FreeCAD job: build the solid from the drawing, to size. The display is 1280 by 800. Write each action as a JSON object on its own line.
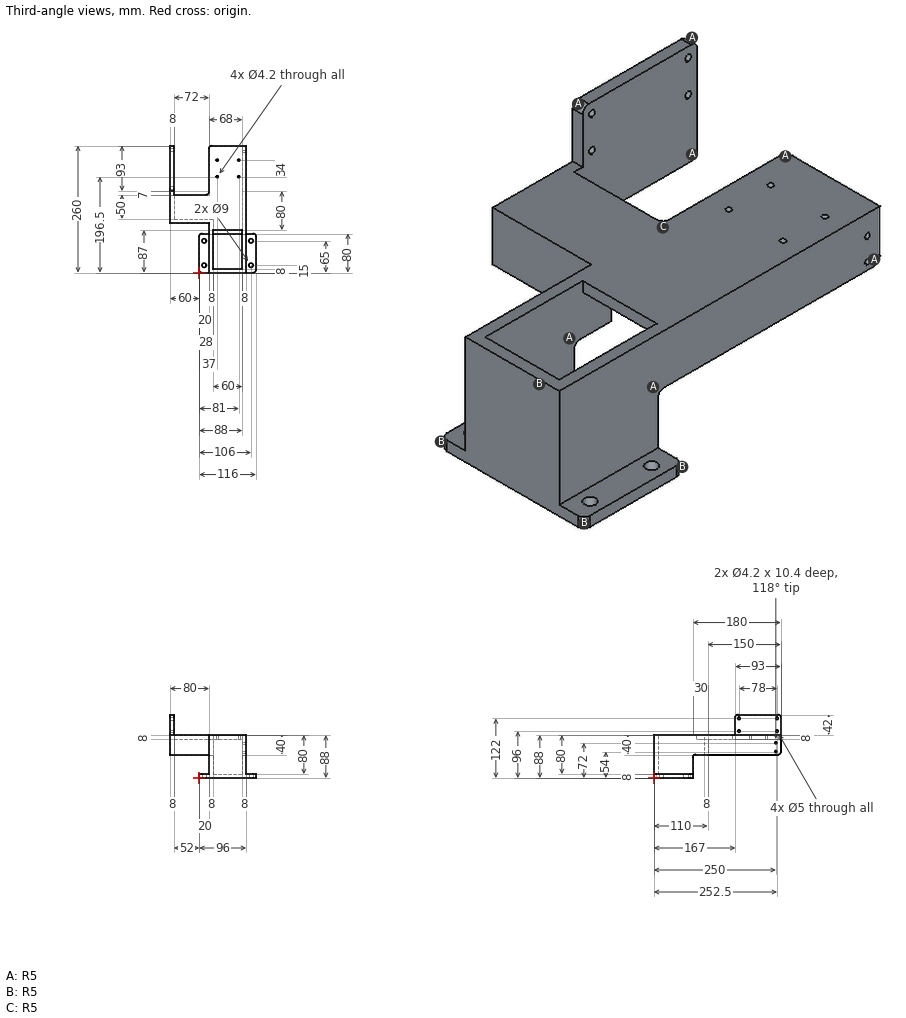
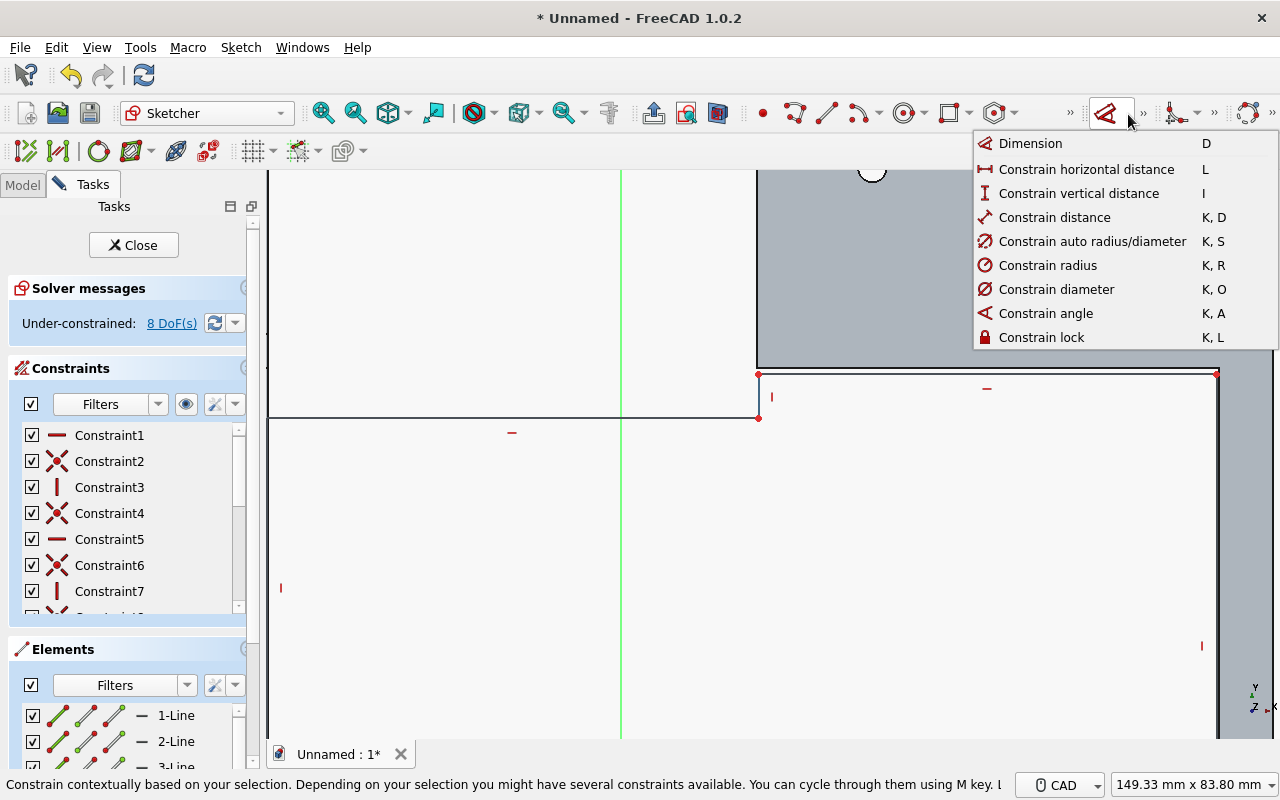
{"action": "left_click", "coordinate": [1126, 193]}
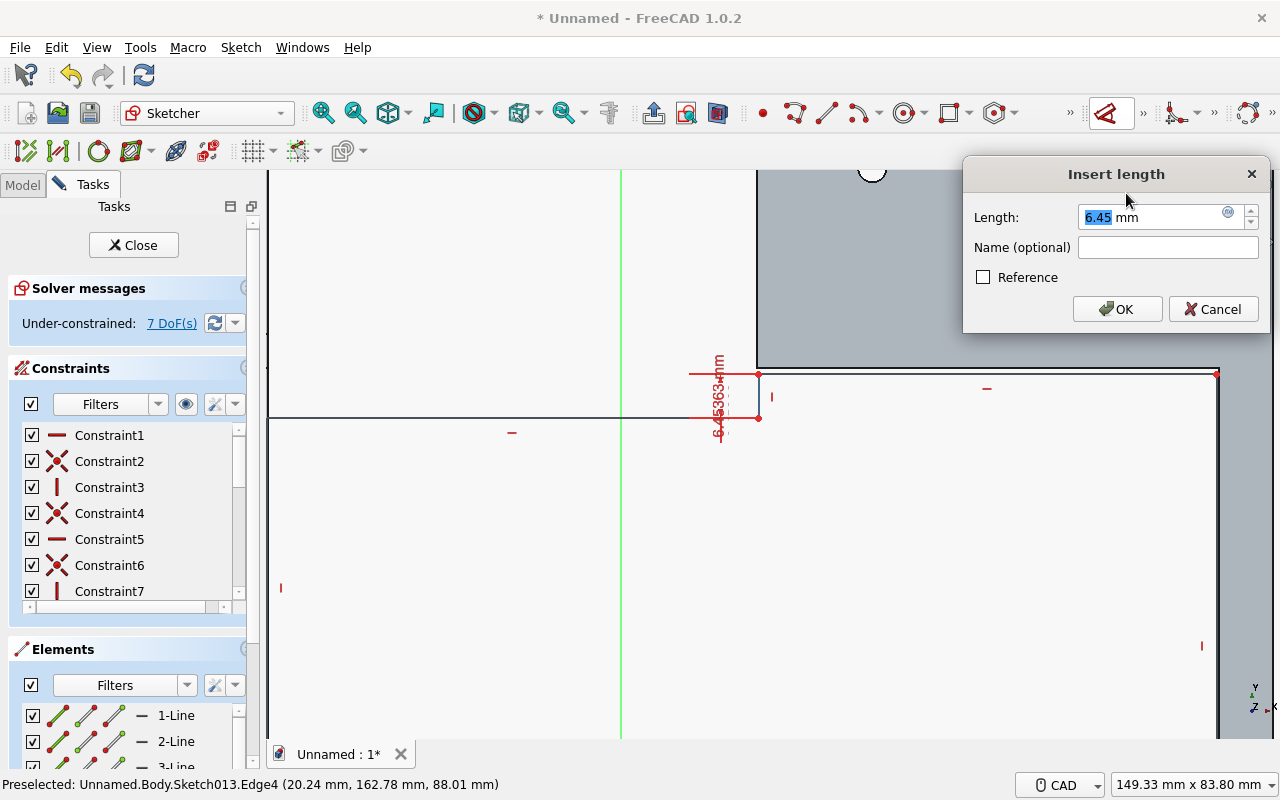
{"action": "type", "text": "7"}
{"action": "key", "text": "Return"}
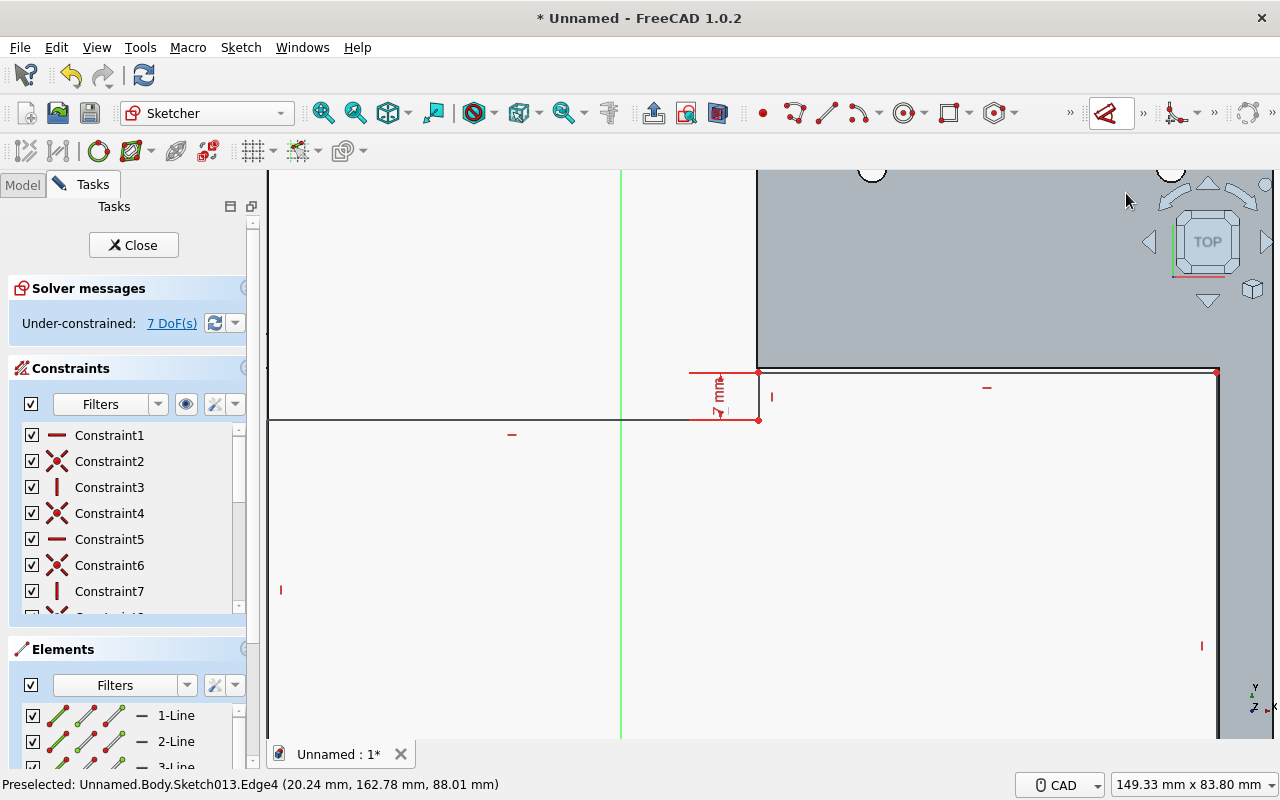
{"action": "scroll", "coordinate": [688, 247], "scroll_direction": "down", "scroll_amount": 6}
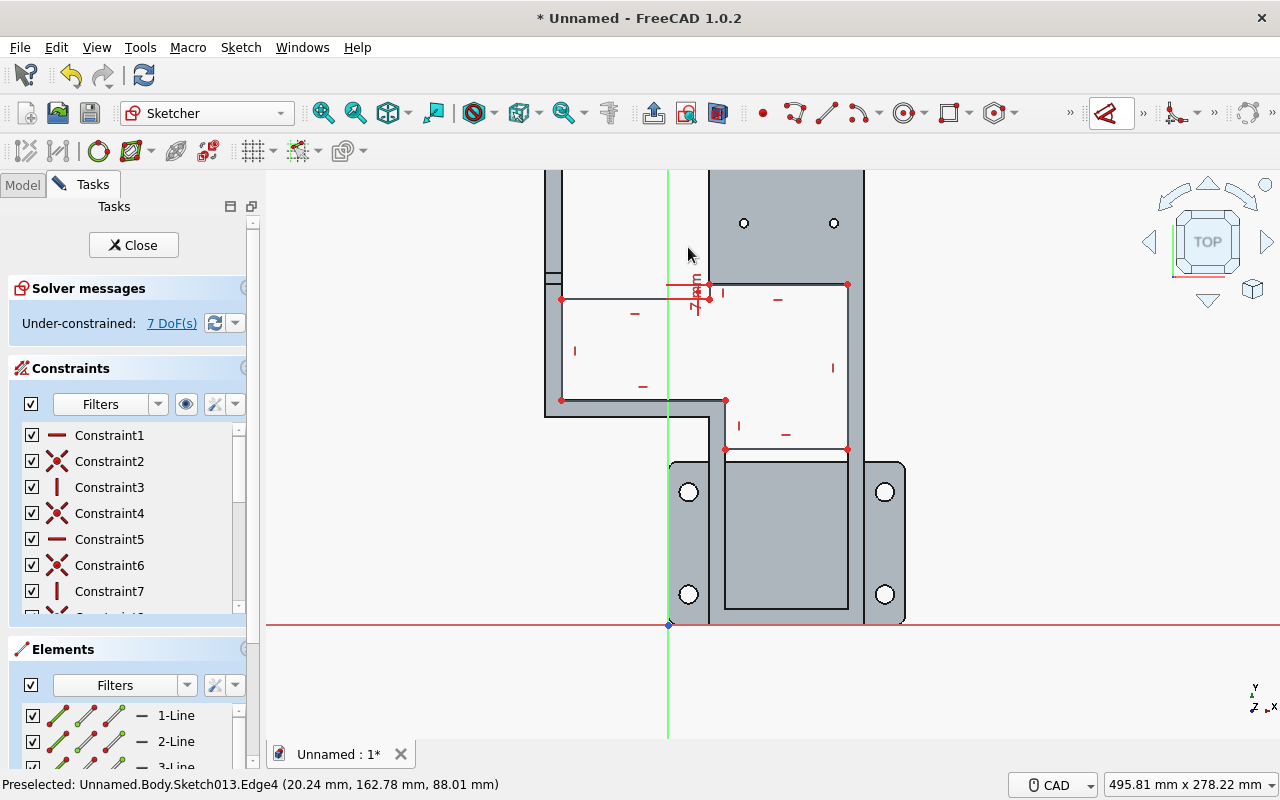
{"action": "left_click", "coordinate": [762, 449]}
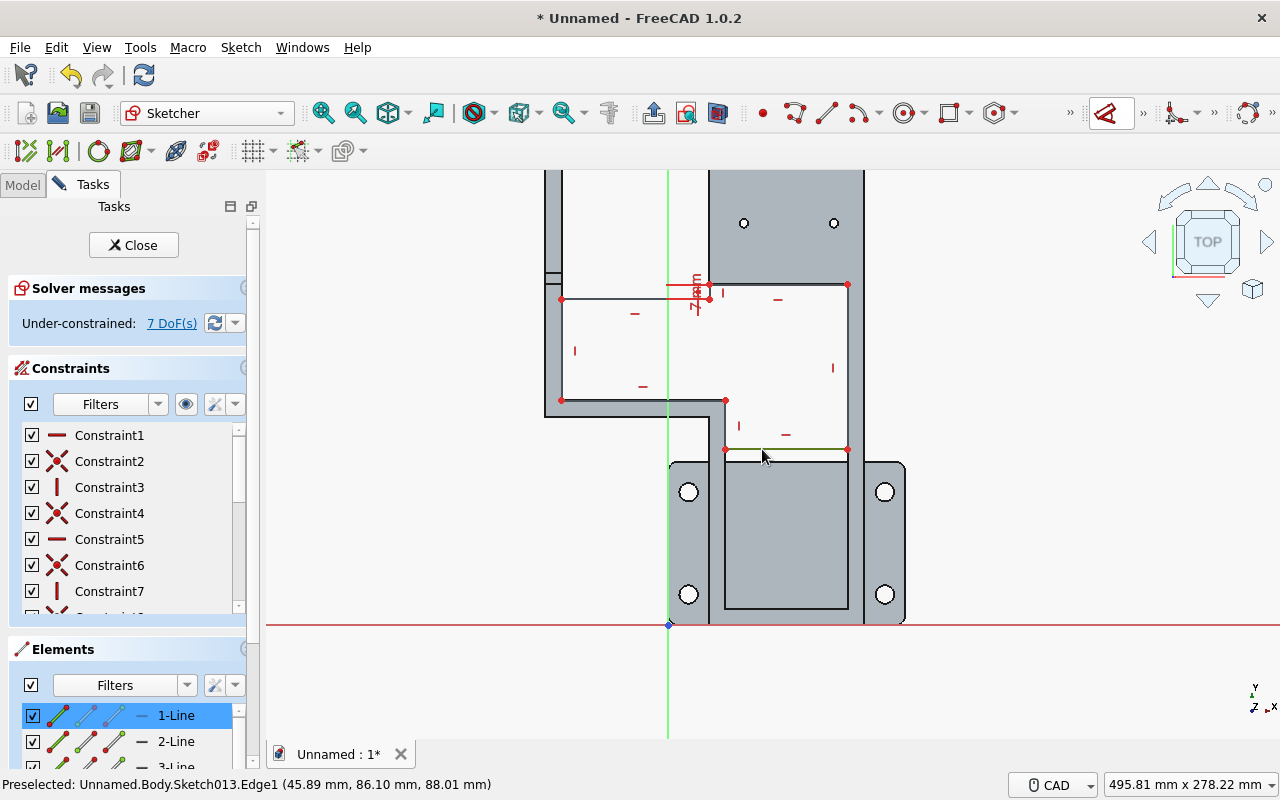
{"action": "left_click", "coordinate": [1128, 114]}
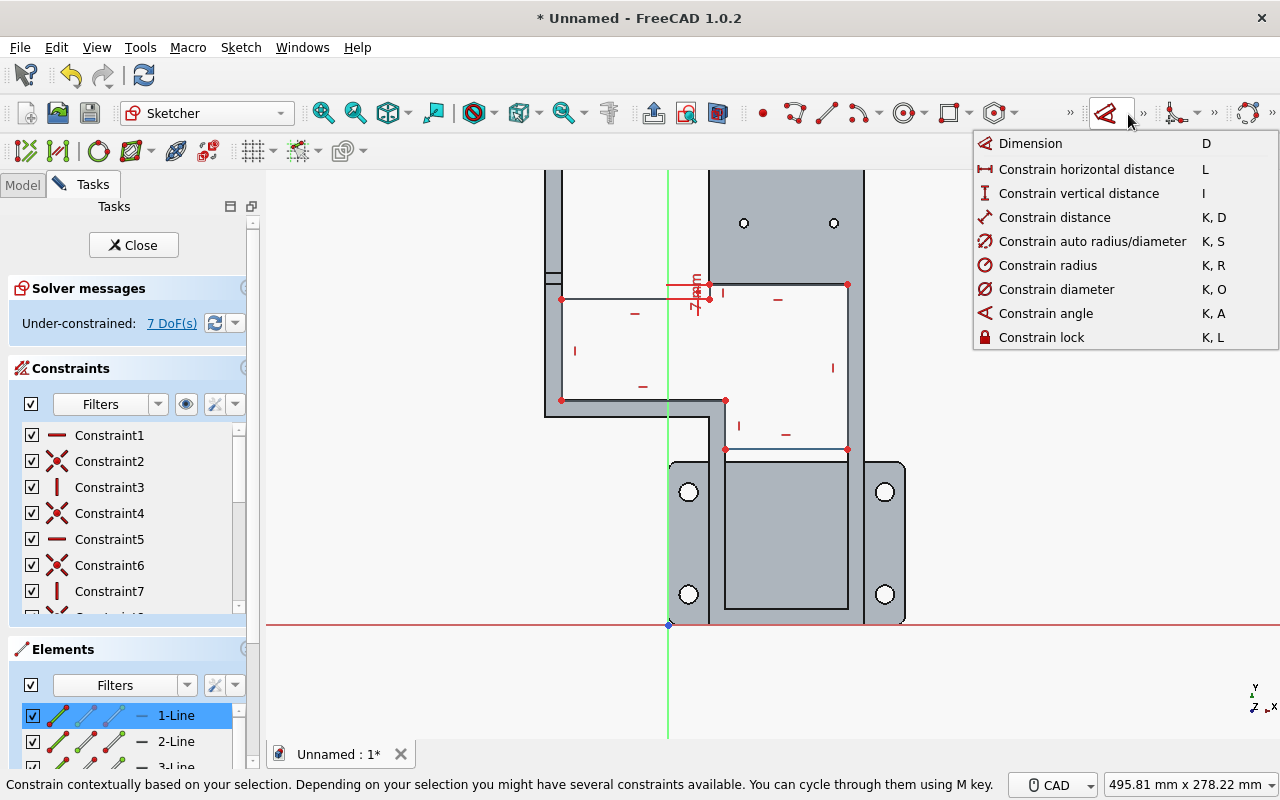
{"action": "left_click", "coordinate": [1126, 169]}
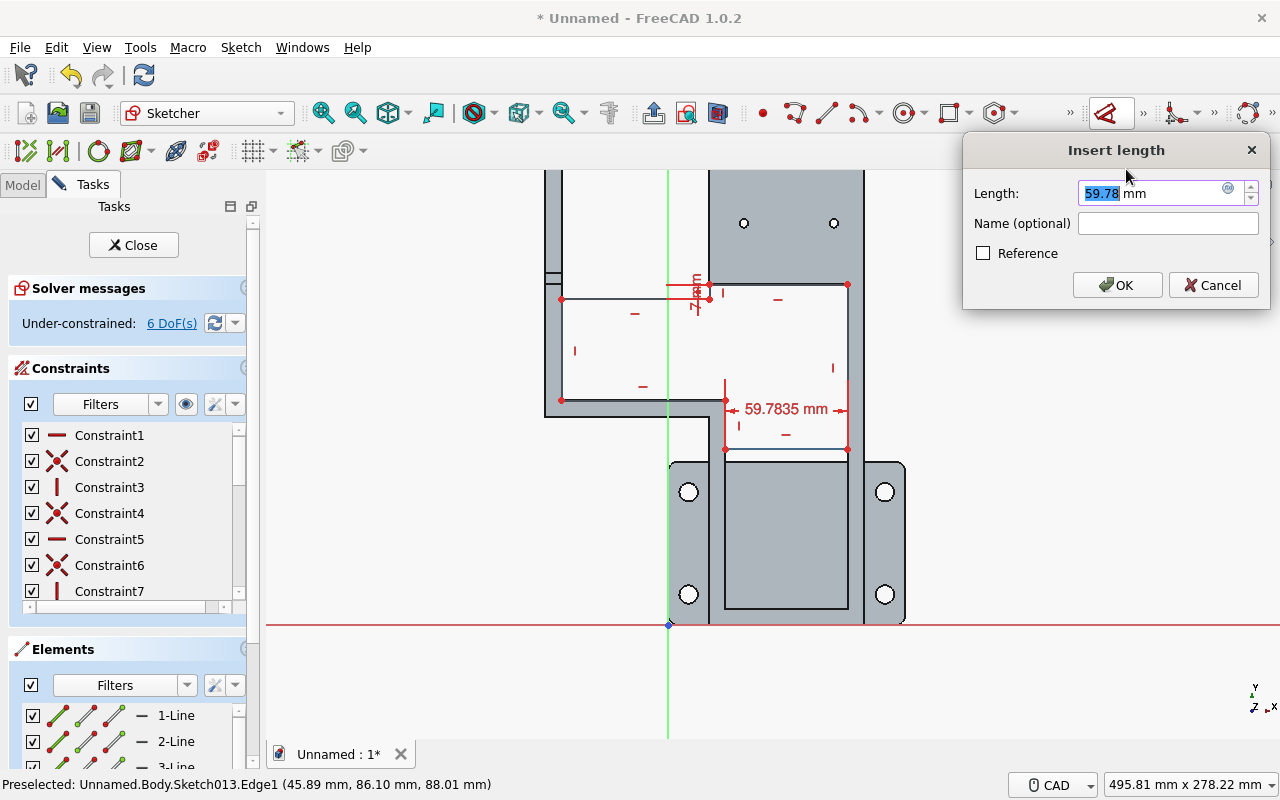
{"action": "type", "text": "60"}
{"action": "key", "text": "Return"}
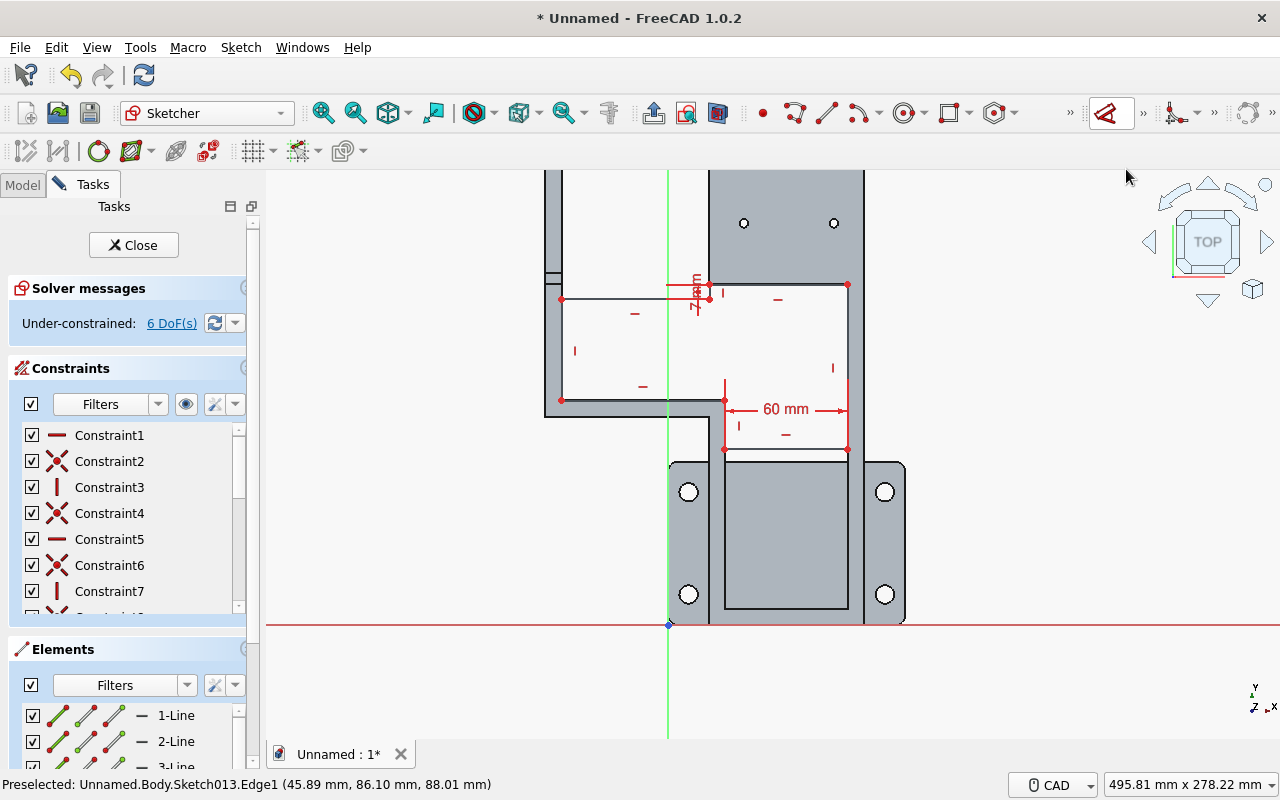
{"action": "left_click", "coordinate": [848, 400]}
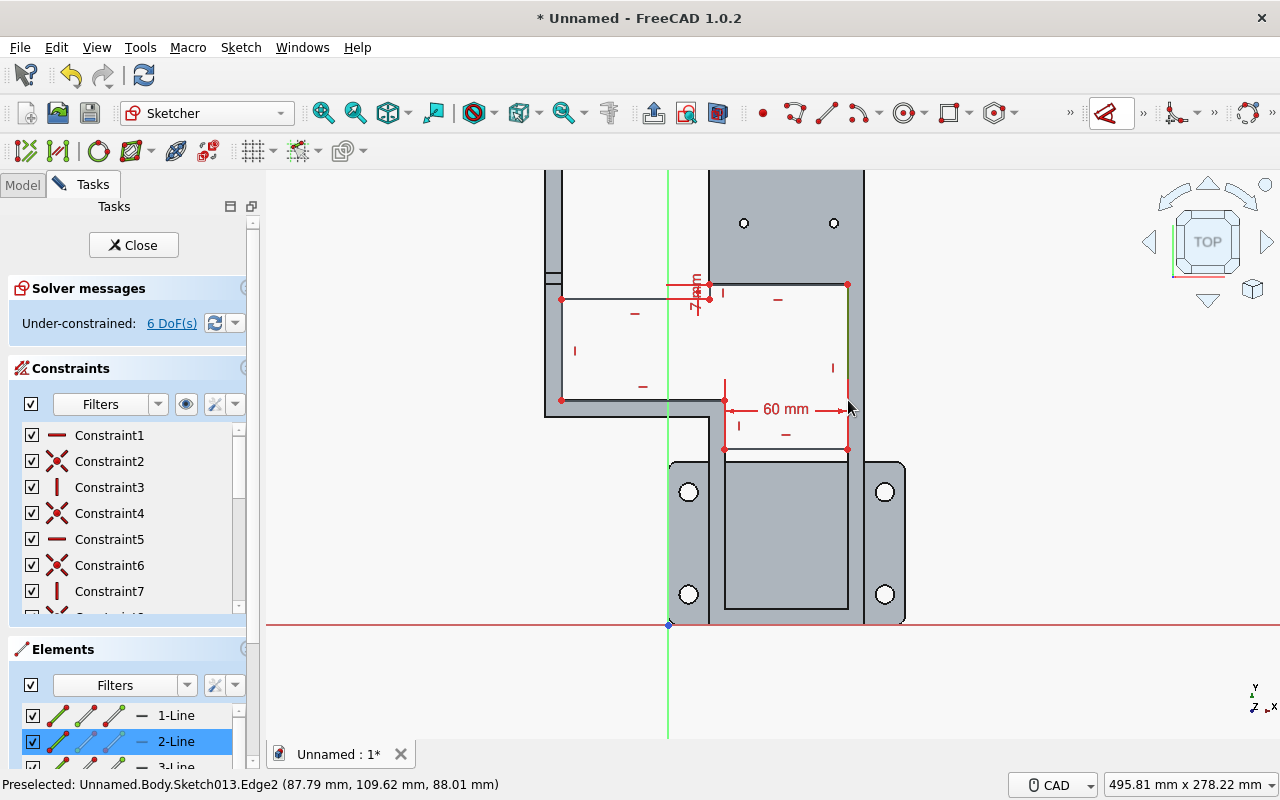
{"action": "left_click", "coordinate": [1128, 114]}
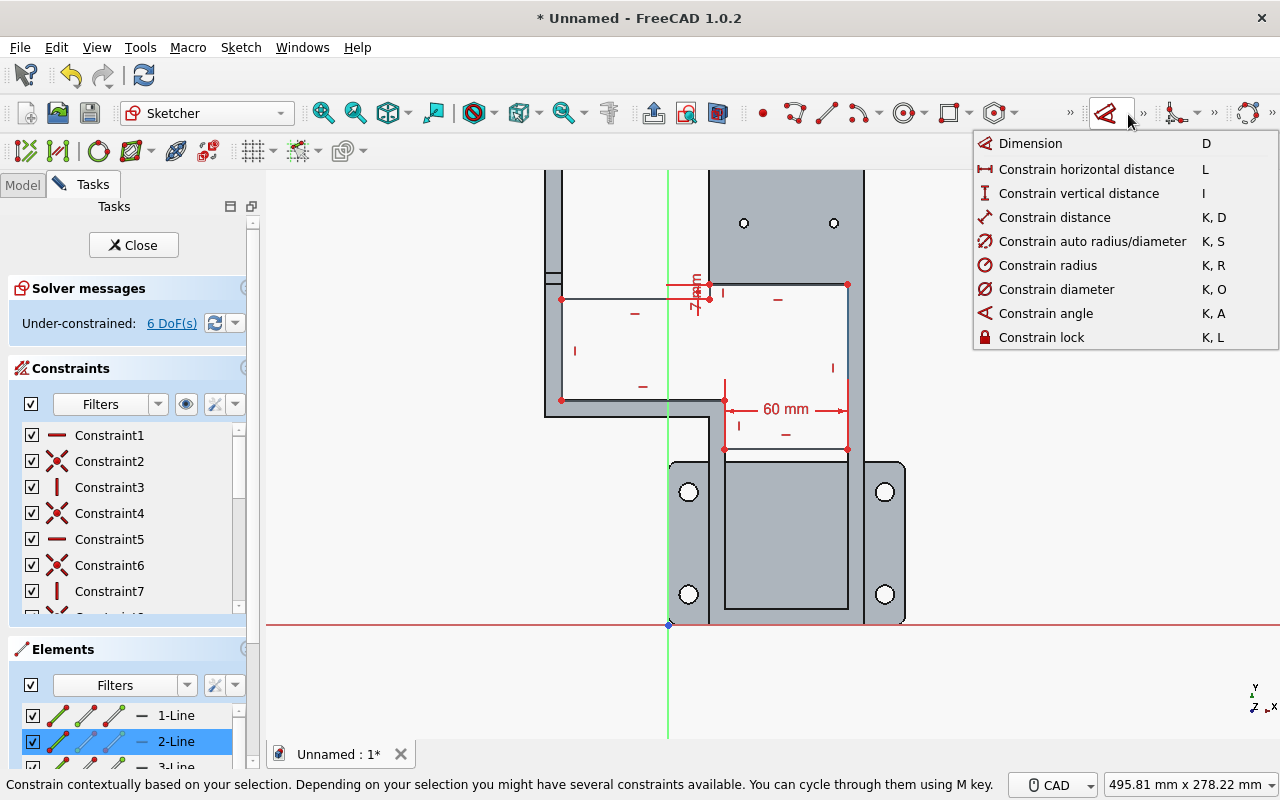
{"action": "left_click", "coordinate": [1126, 193]}